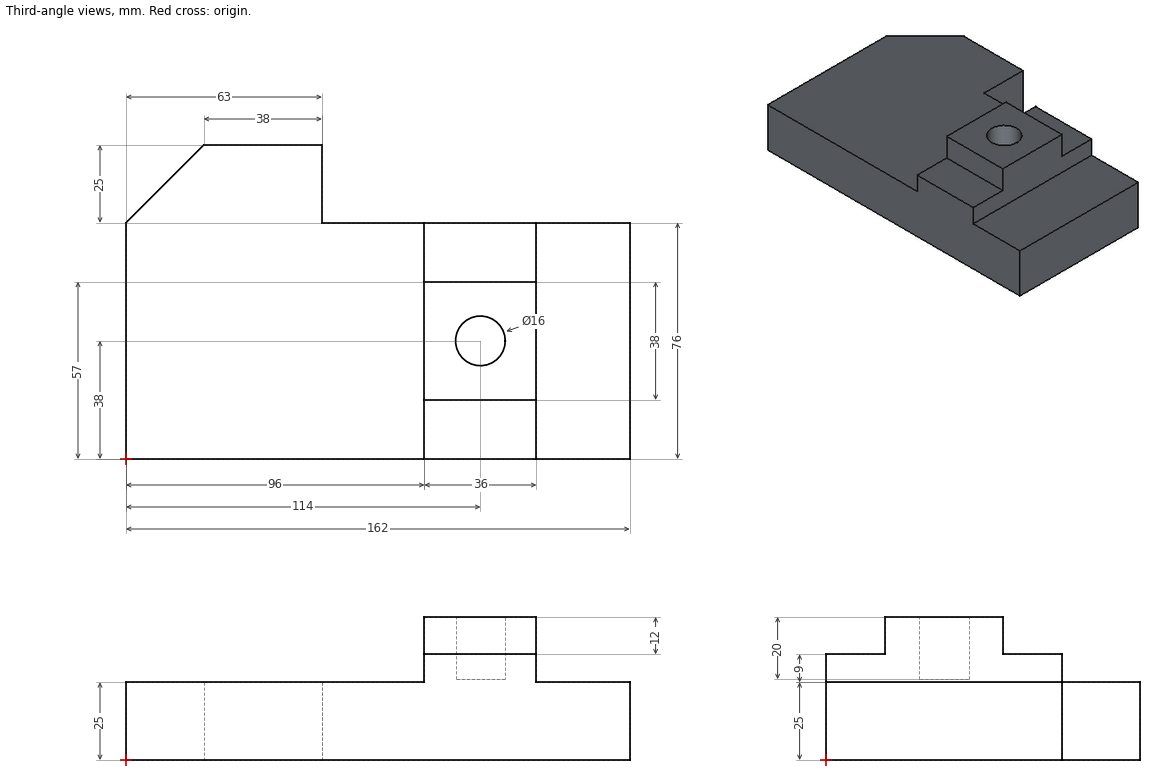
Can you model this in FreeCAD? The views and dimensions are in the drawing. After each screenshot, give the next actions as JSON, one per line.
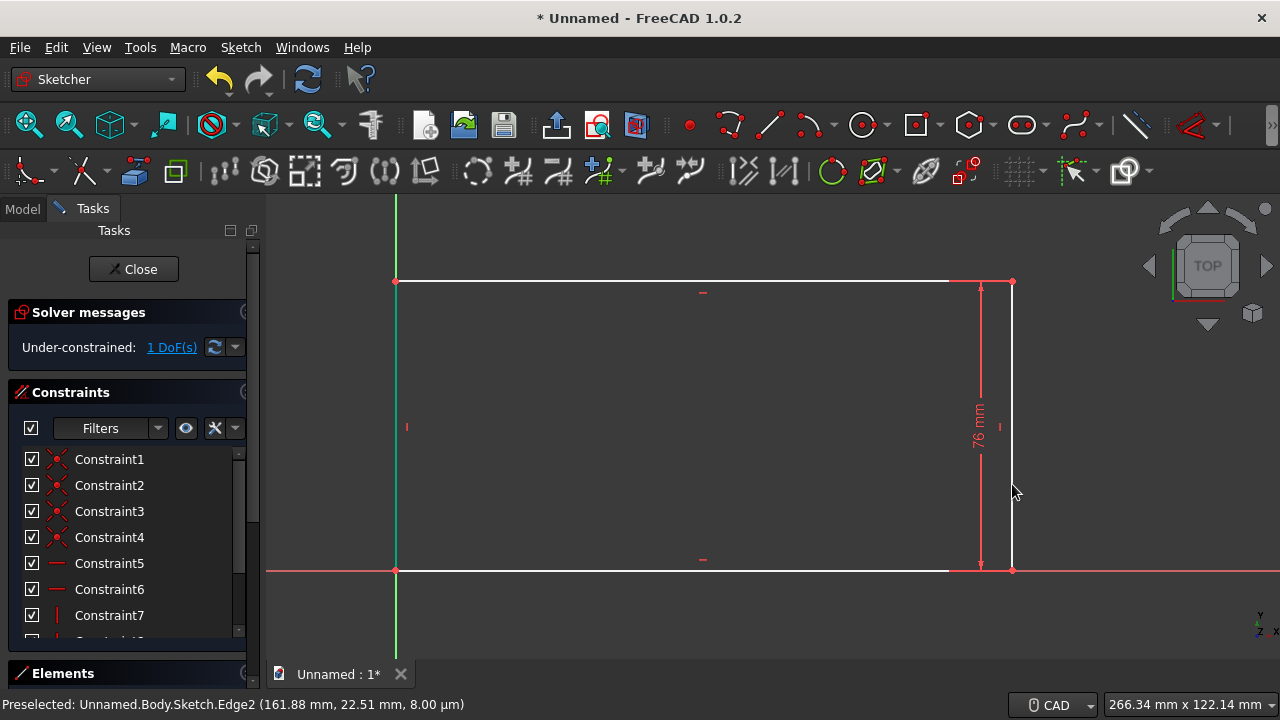
{"action": "left_click", "coordinate": [581, 571]}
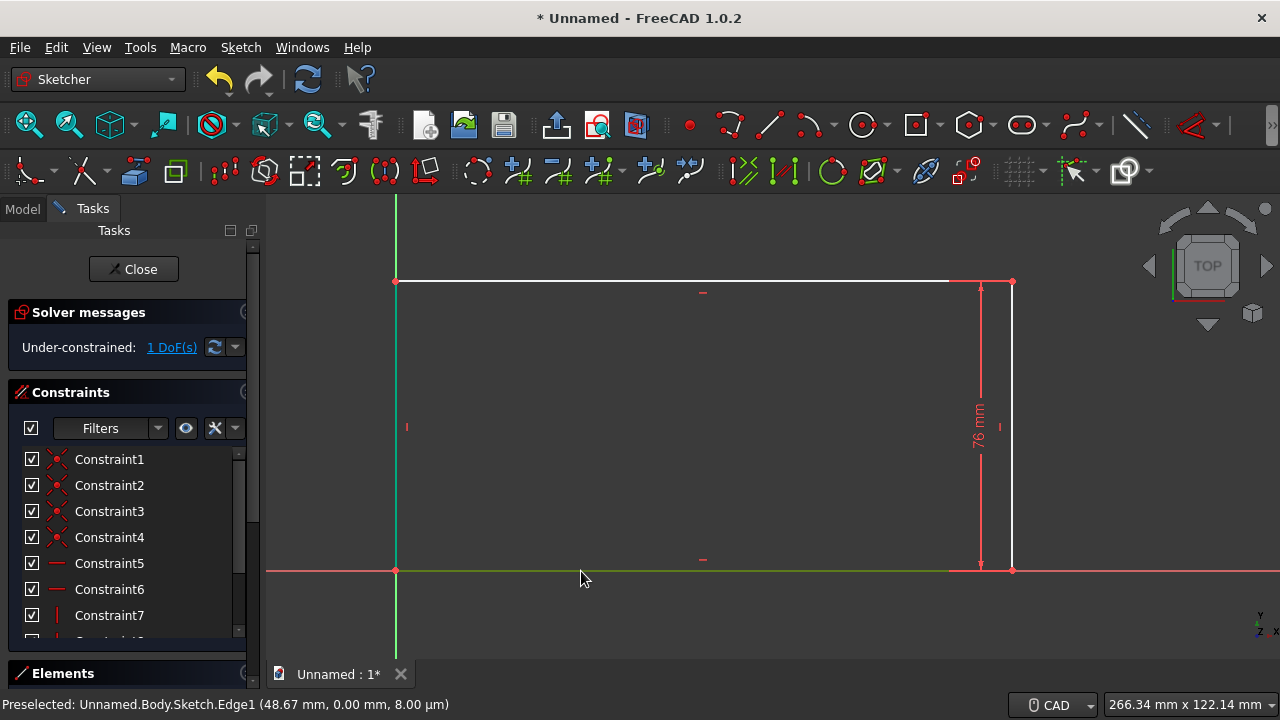
{"action": "key", "text": "l"}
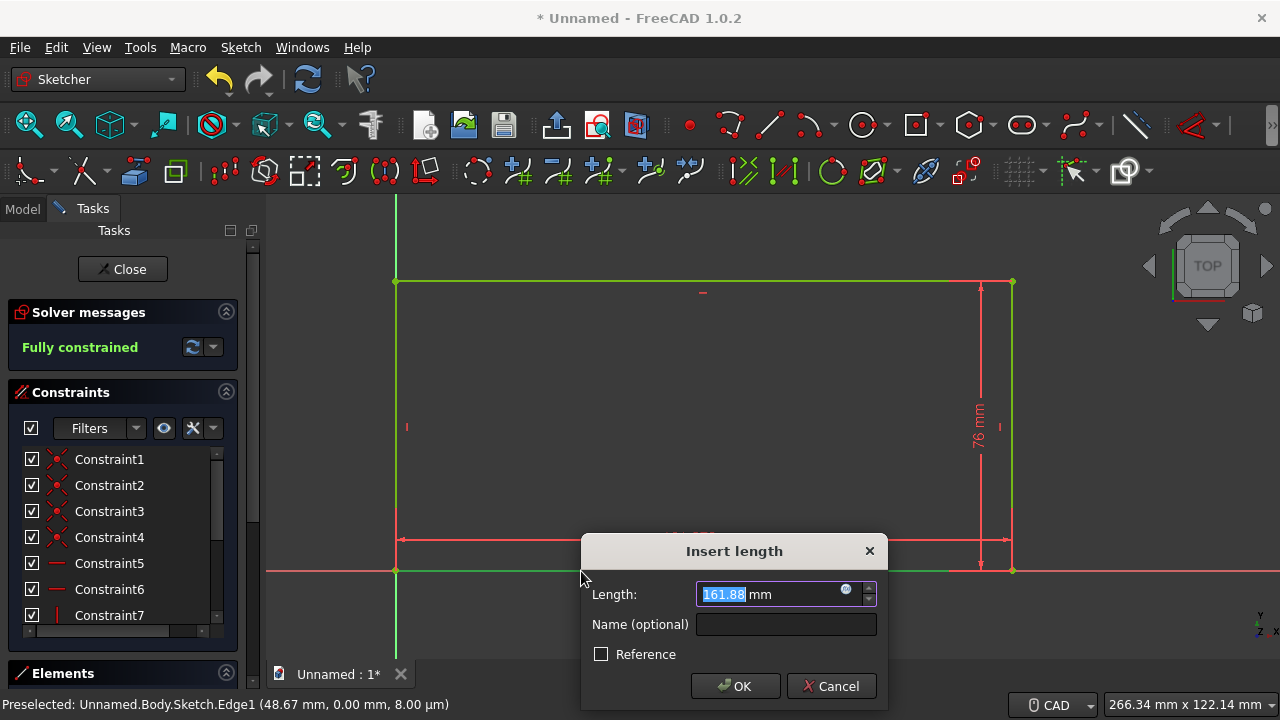
{"action": "type", "text": "162"}
{"action": "key", "text": "Return"}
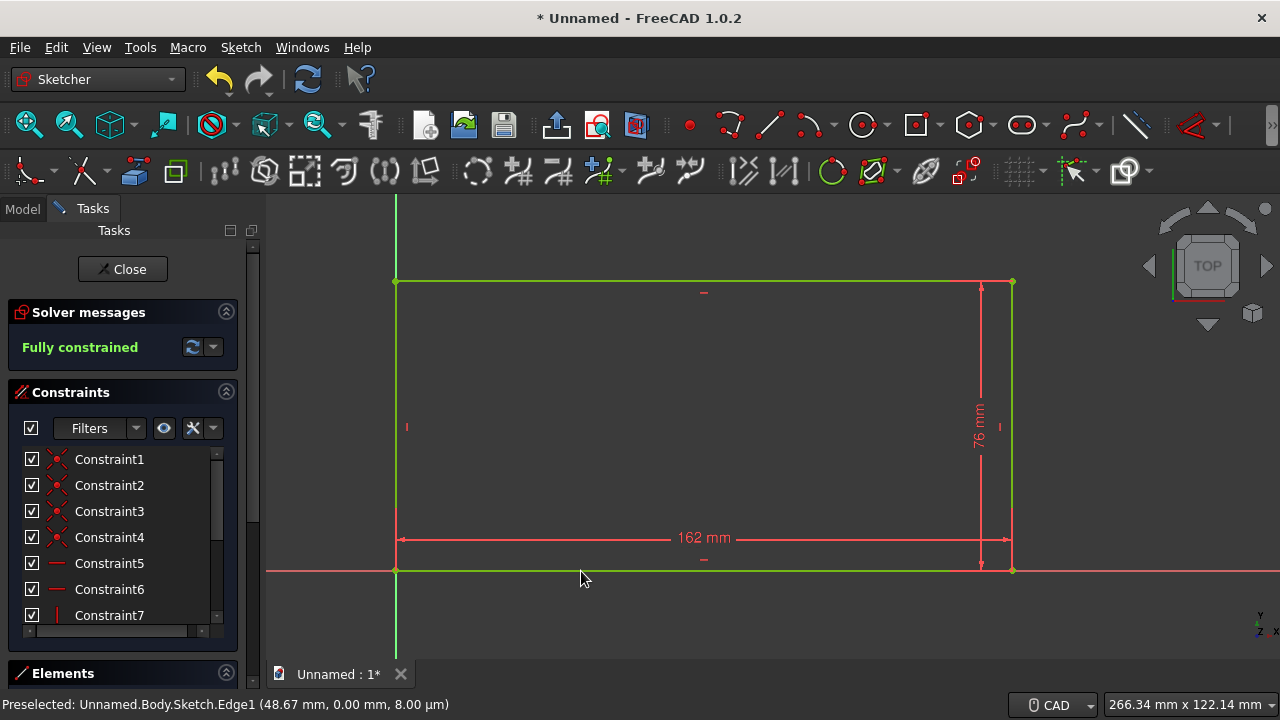
{"action": "left_click", "coordinate": [123, 269]}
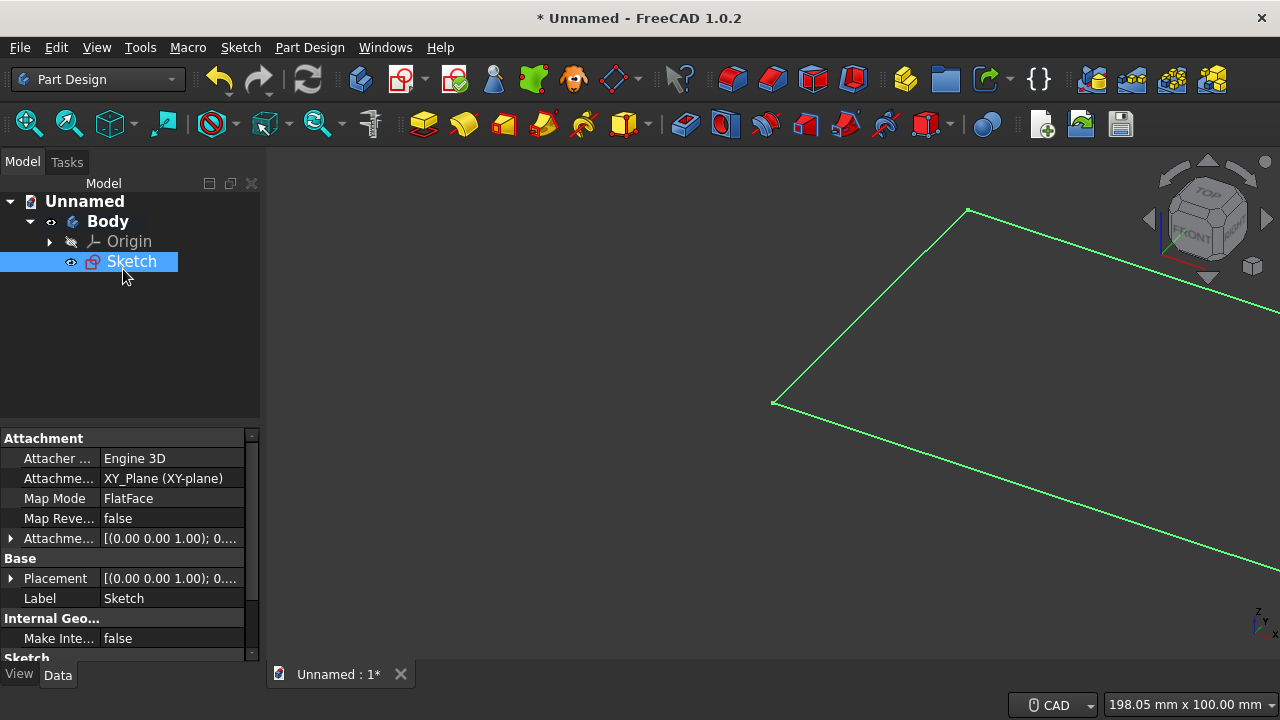
{"action": "left_click", "coordinate": [424, 124]}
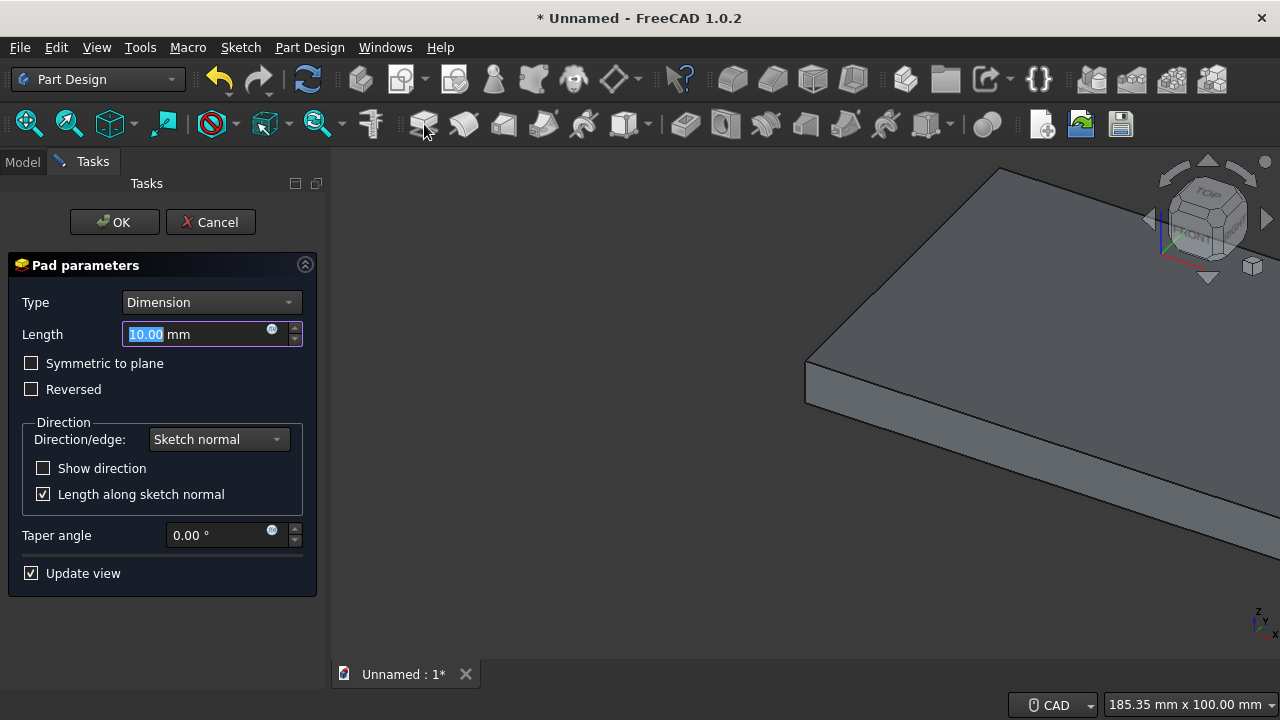
{"action": "type", "text": "25"}
{"action": "key", "text": "Tab"}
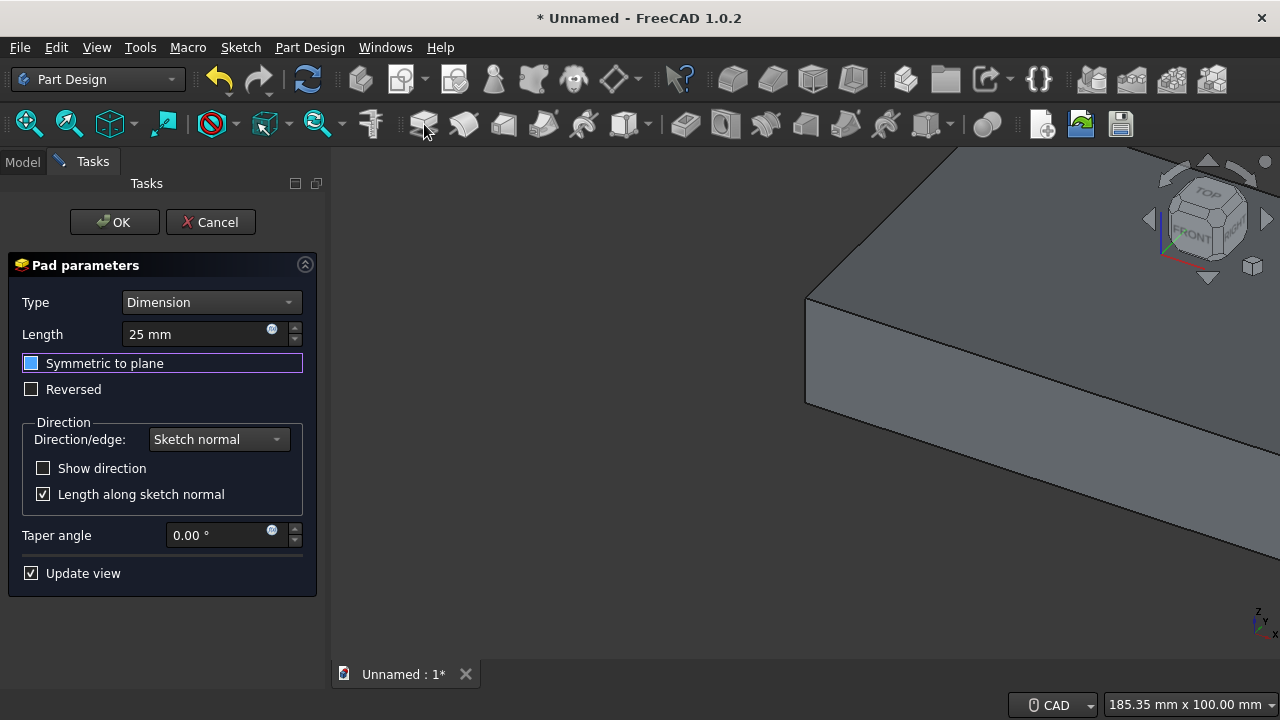
{"action": "left_click", "coordinate": [115, 222]}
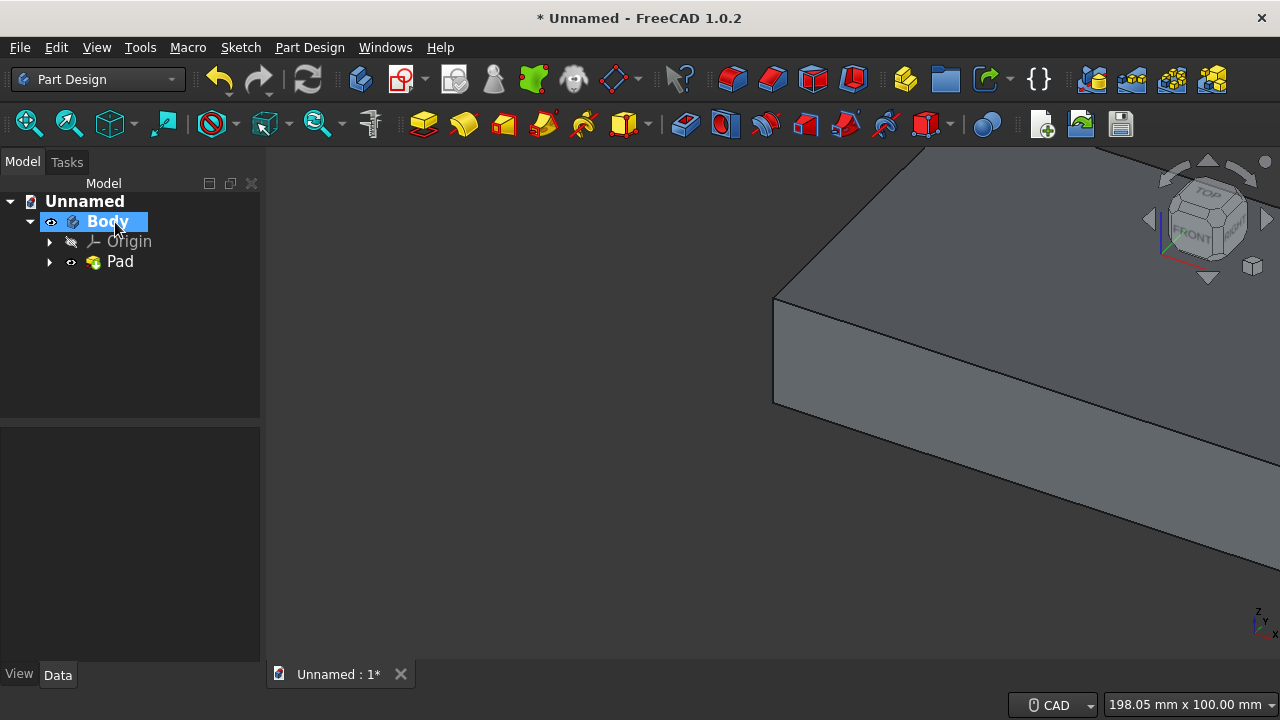
{"action": "key", "text": "v f"}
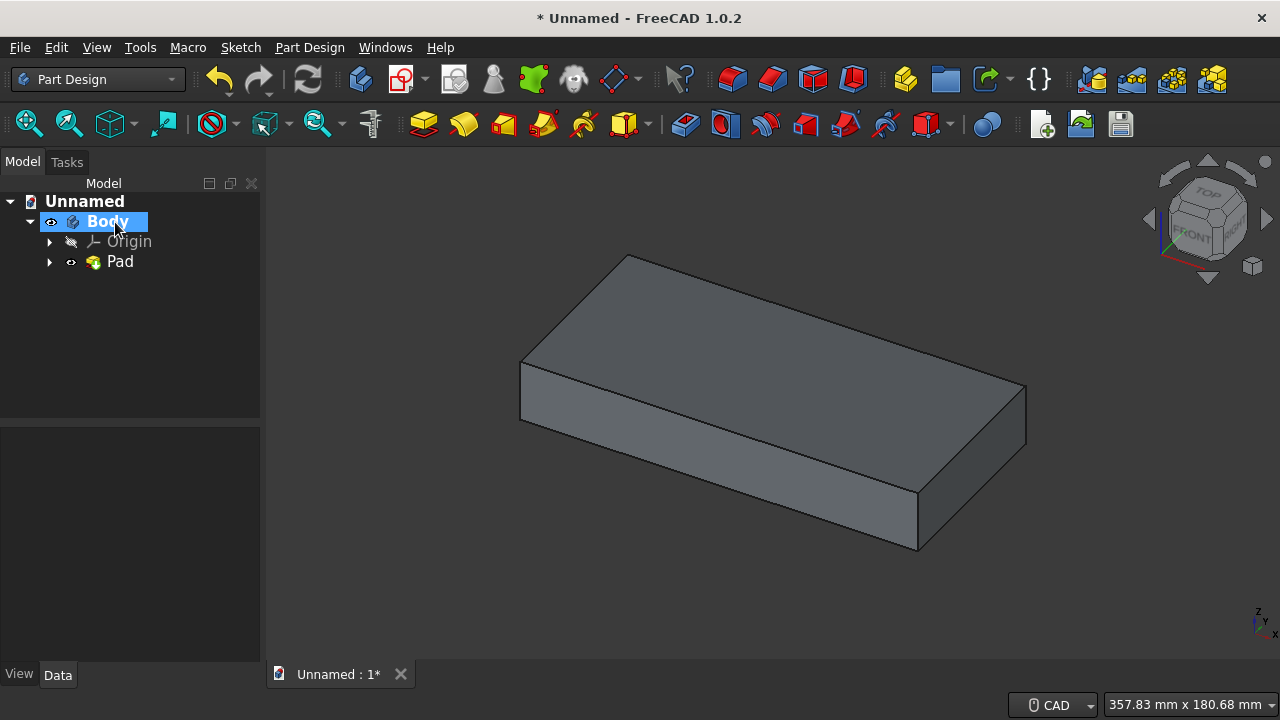
{"action": "left_click", "coordinate": [830, 392]}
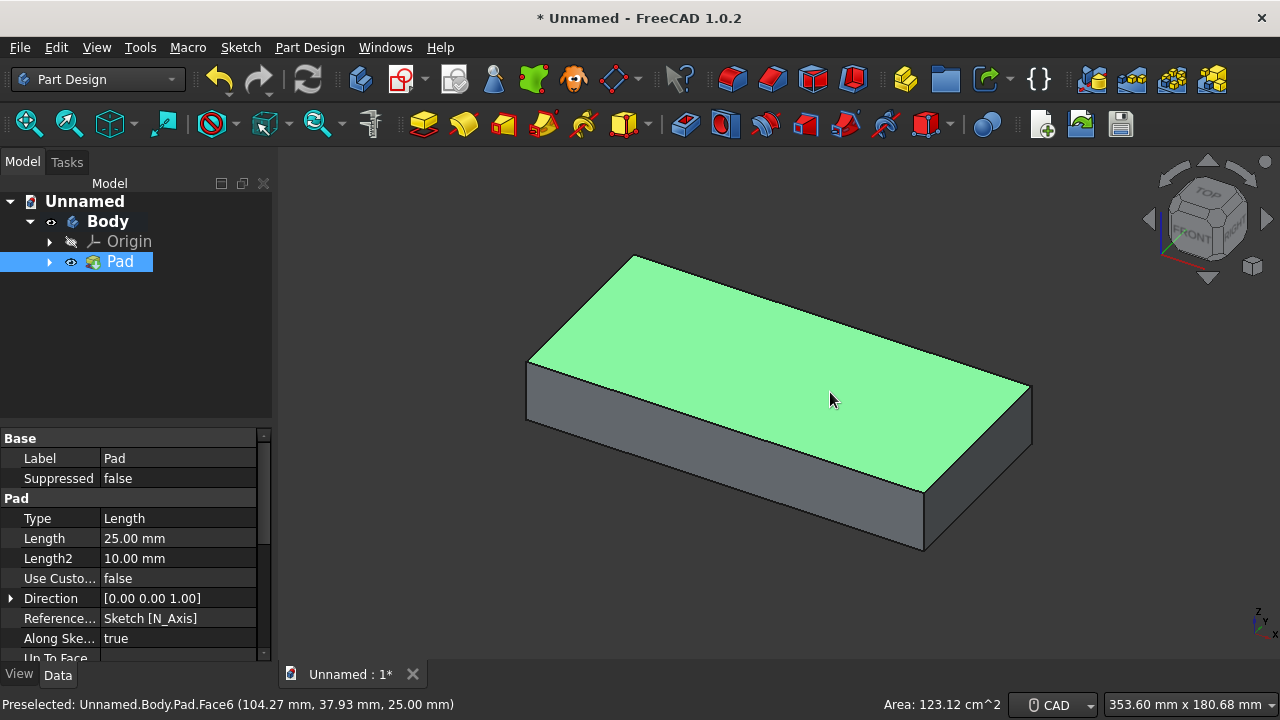
{"action": "left_click", "coordinate": [402, 80]}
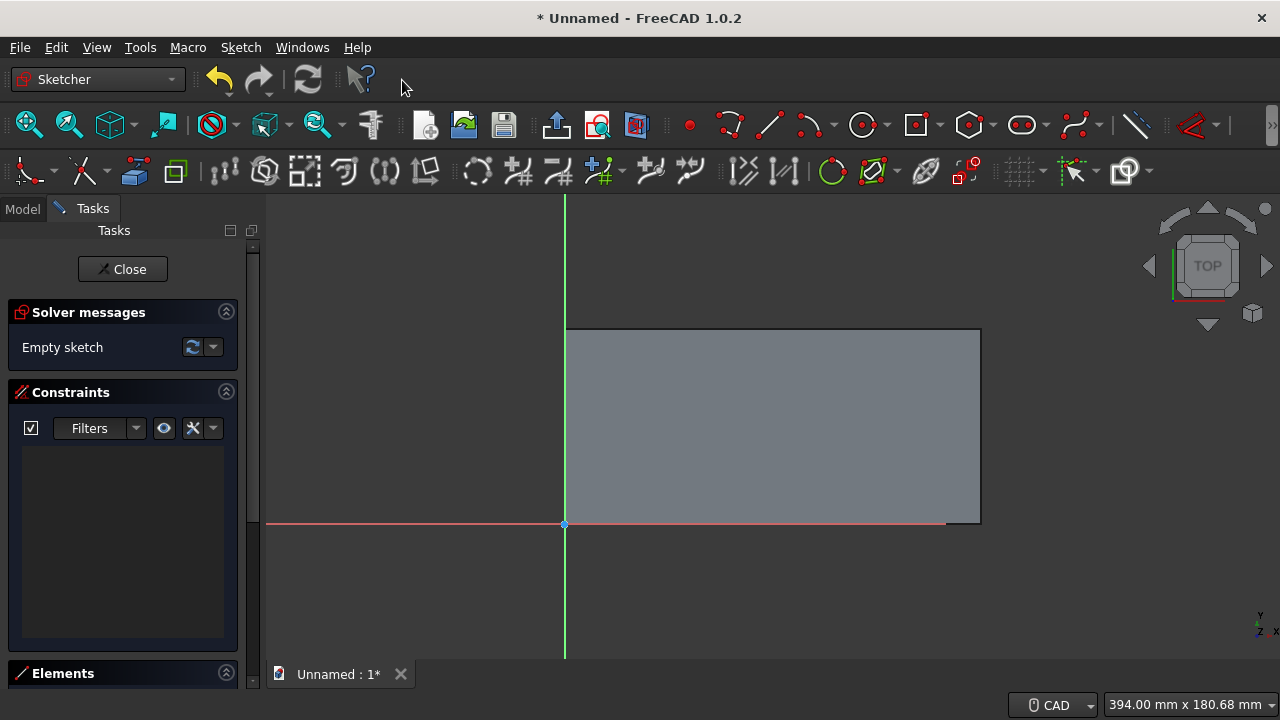
{"action": "key", "text": "g m"}